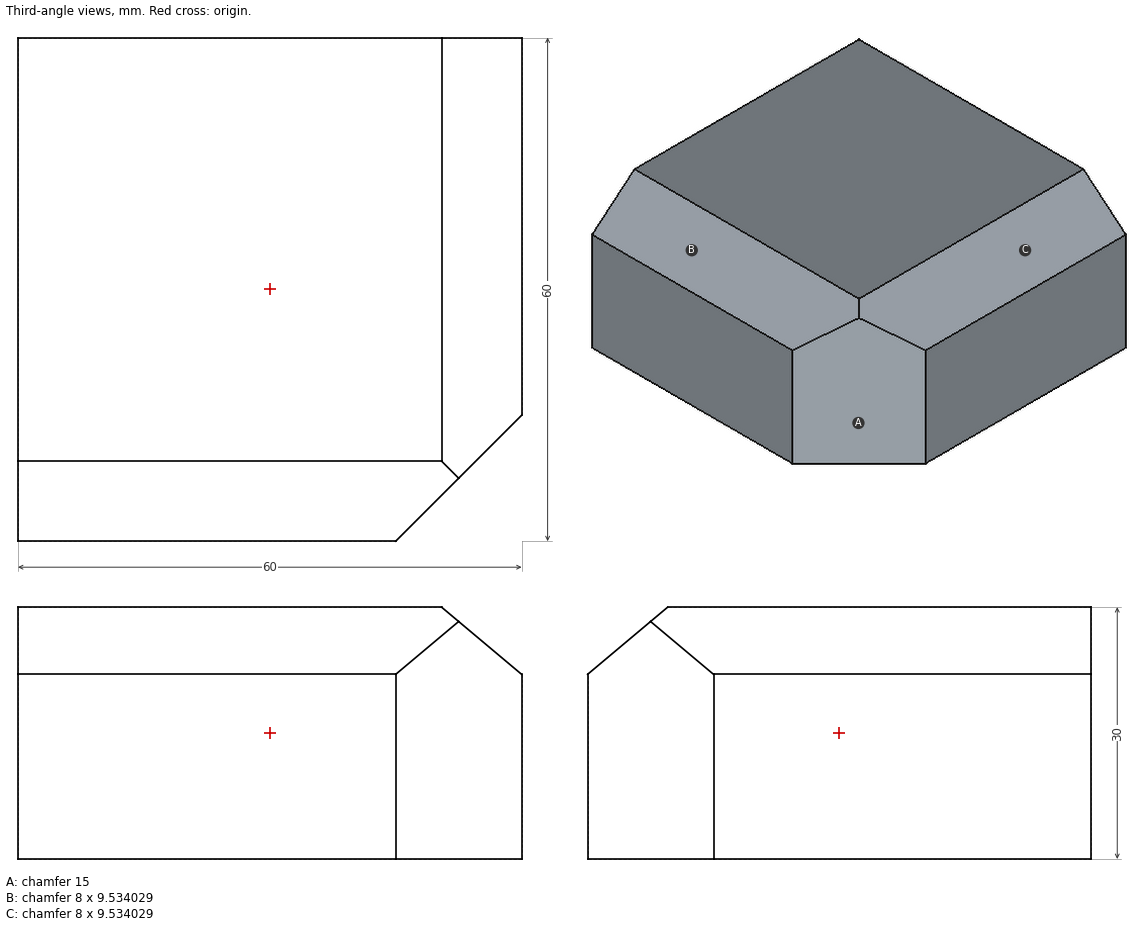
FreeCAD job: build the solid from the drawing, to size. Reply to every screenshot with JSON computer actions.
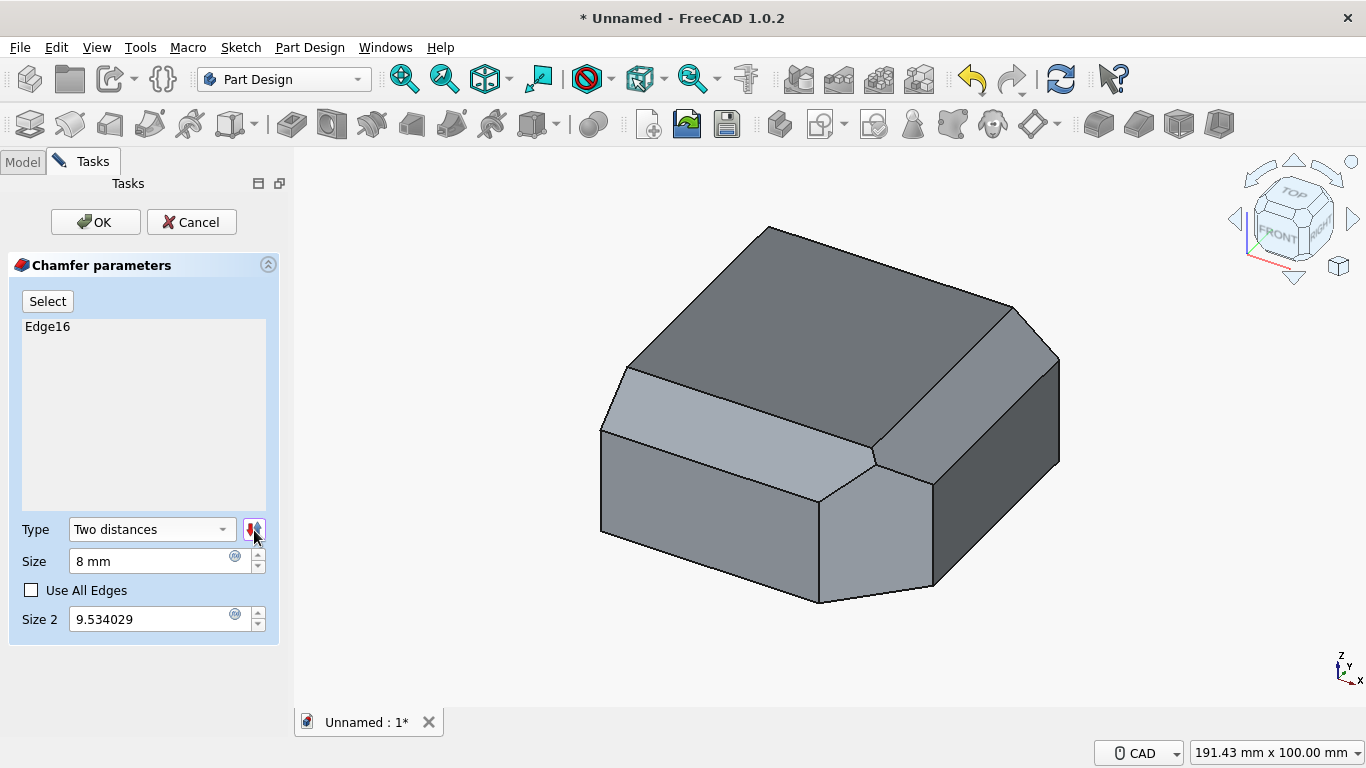
{"action": "left_click", "coordinate": [96, 222]}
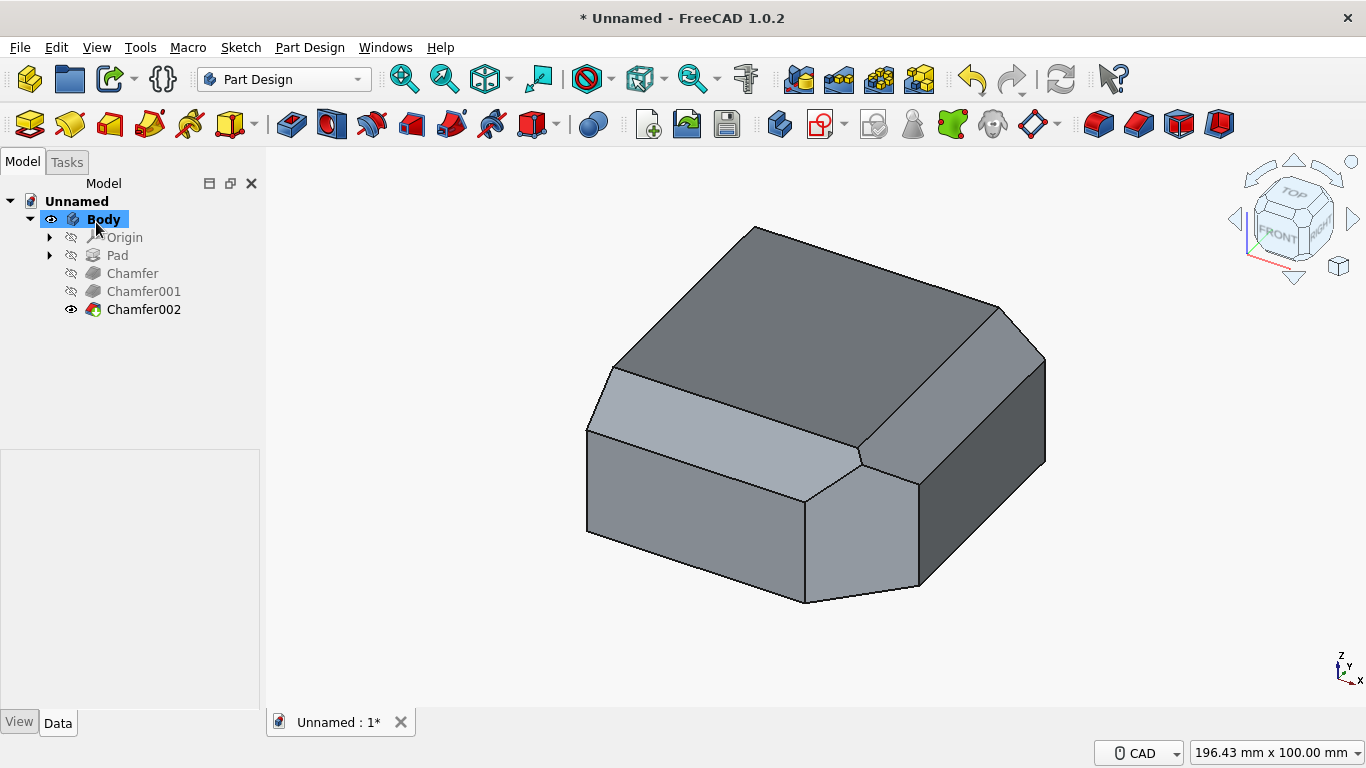
{"action": "key", "text": "0"}